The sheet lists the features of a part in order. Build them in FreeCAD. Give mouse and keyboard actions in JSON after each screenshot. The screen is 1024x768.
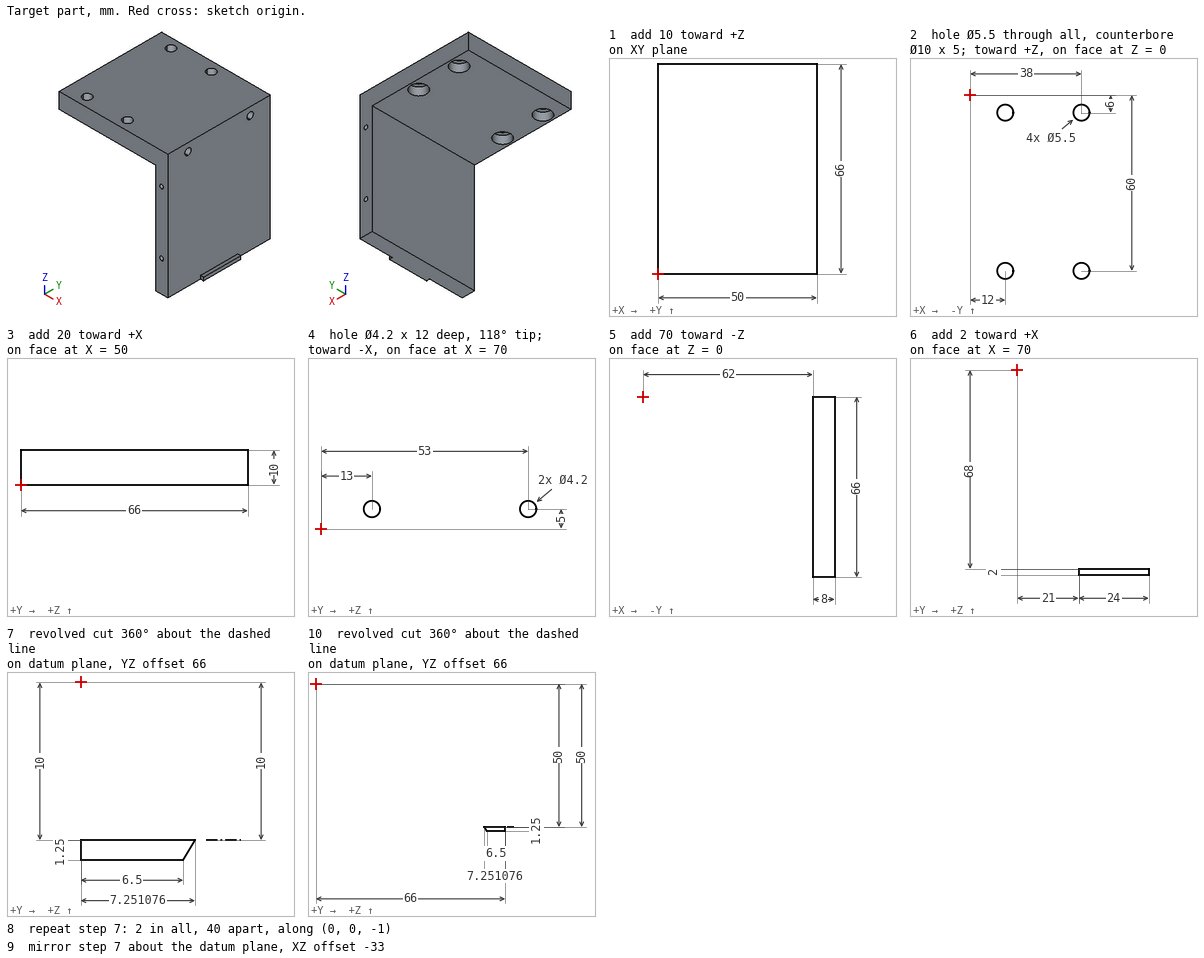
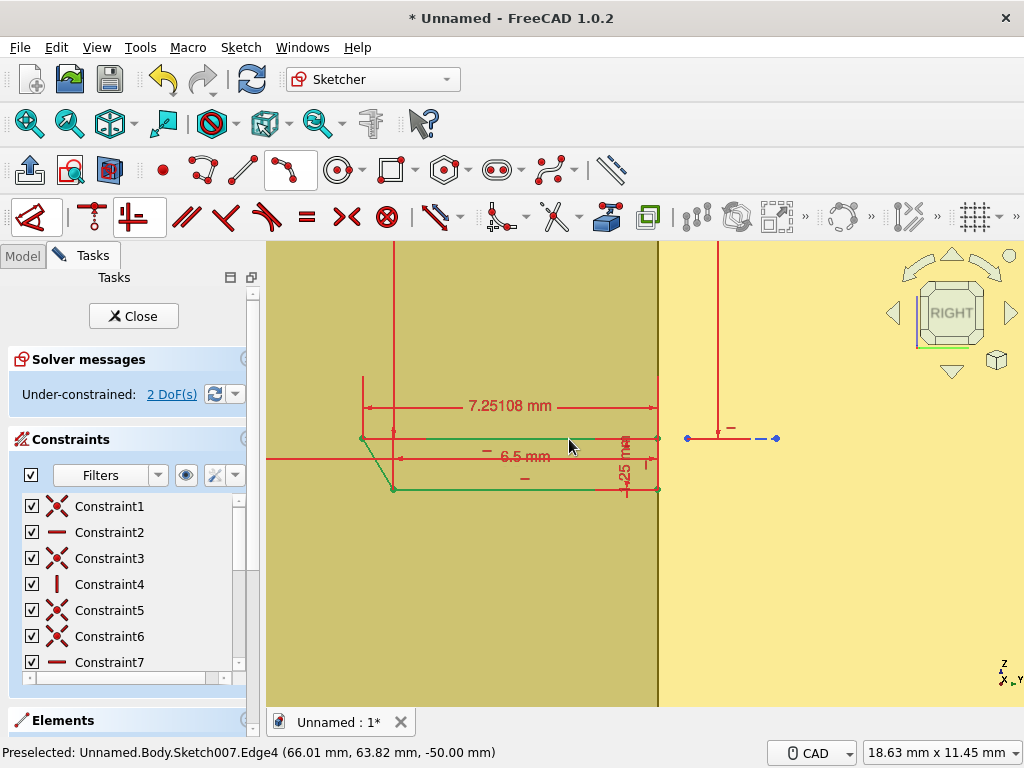
{"action": "left_click", "coordinate": [134, 316]}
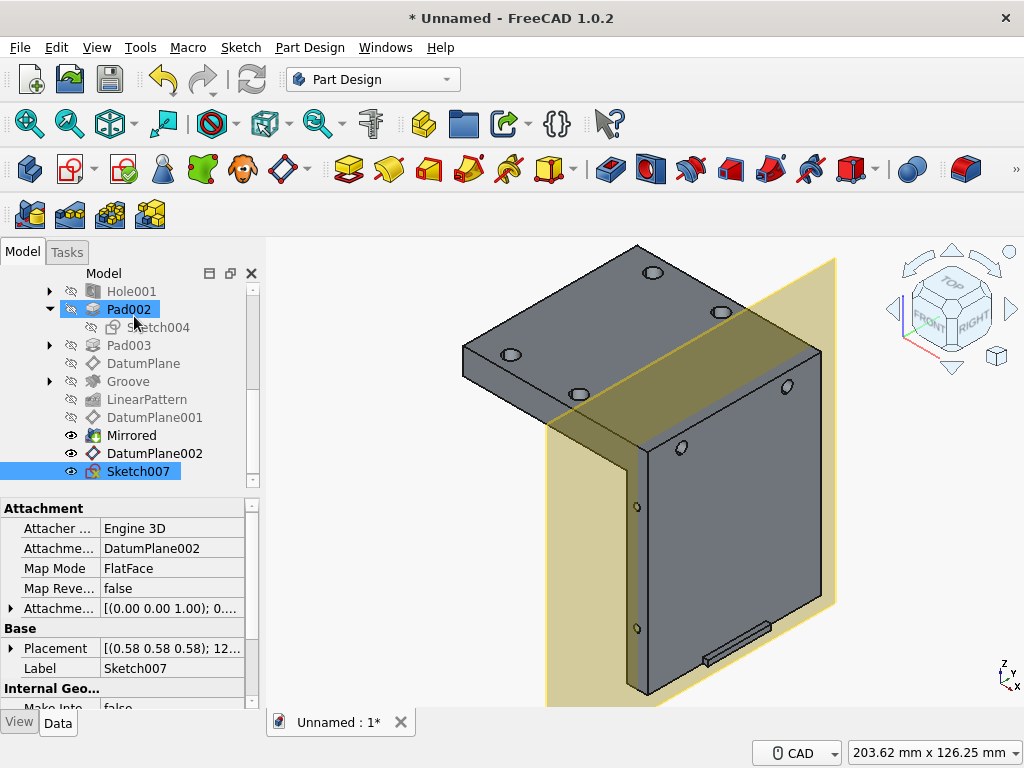
{"action": "left_click", "coordinate": [692, 170]}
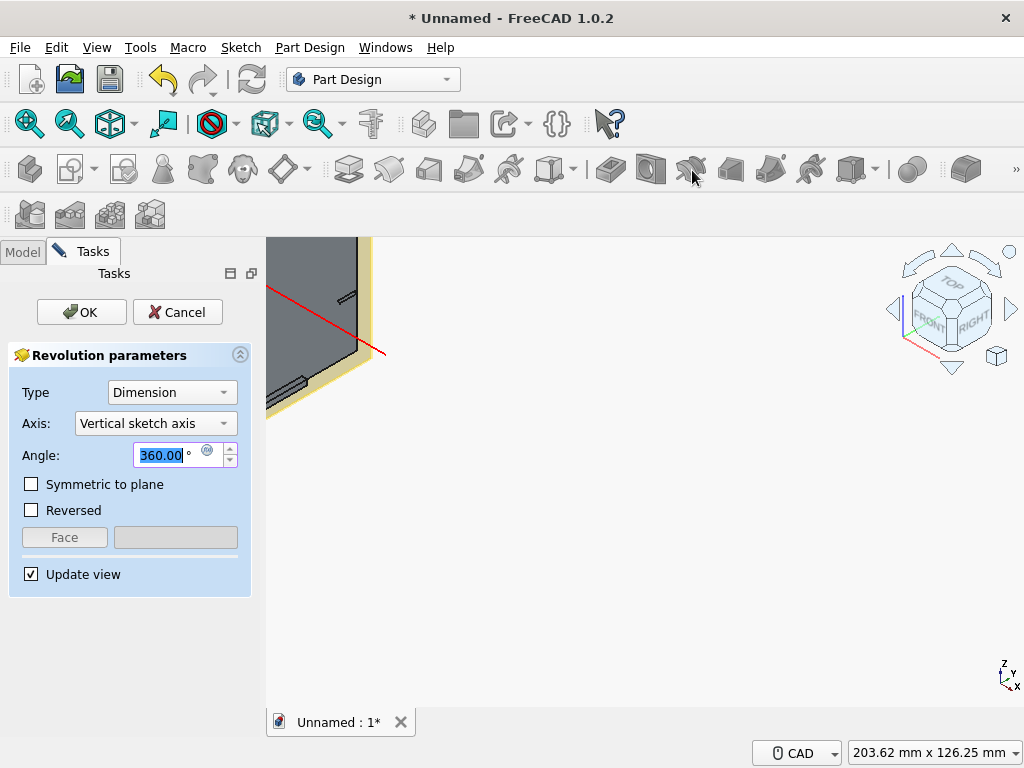
{"action": "left_click", "coordinate": [156, 424]}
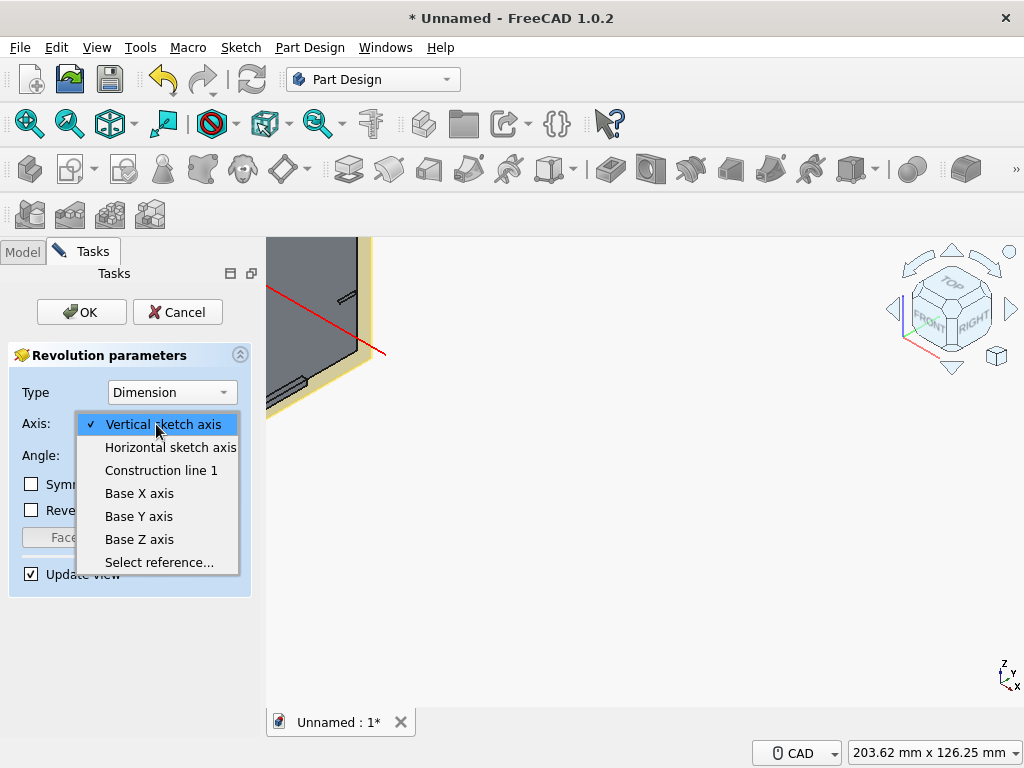
{"action": "left_click", "coordinate": [156, 470]}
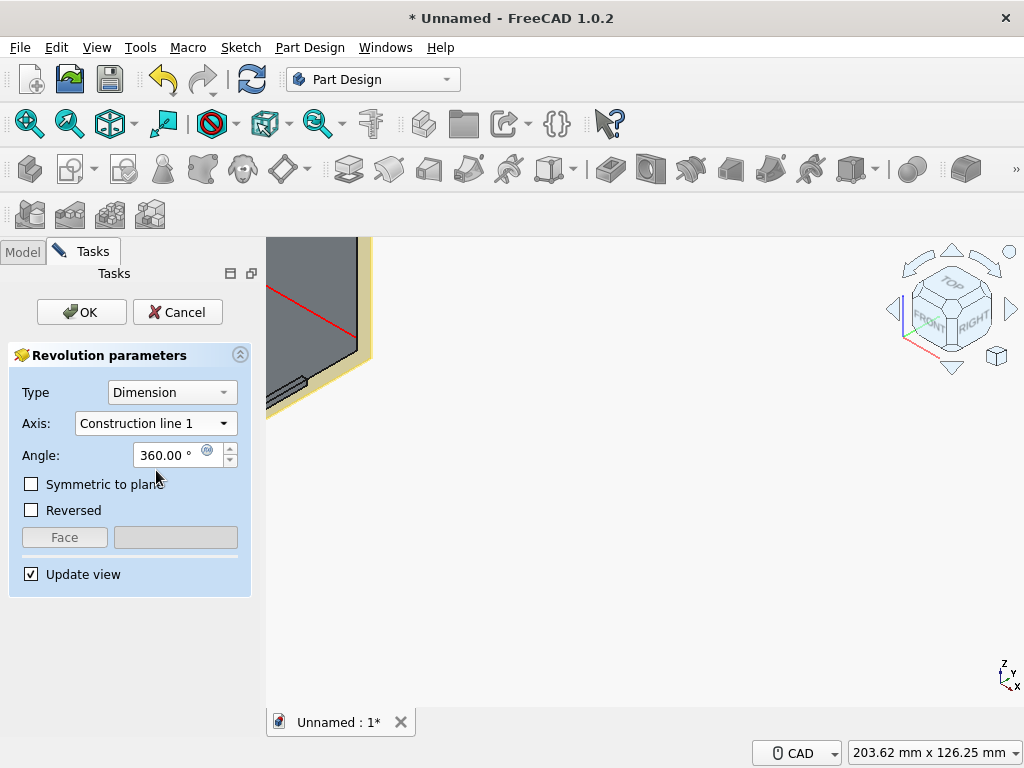
{"action": "left_click", "coordinate": [82, 312]}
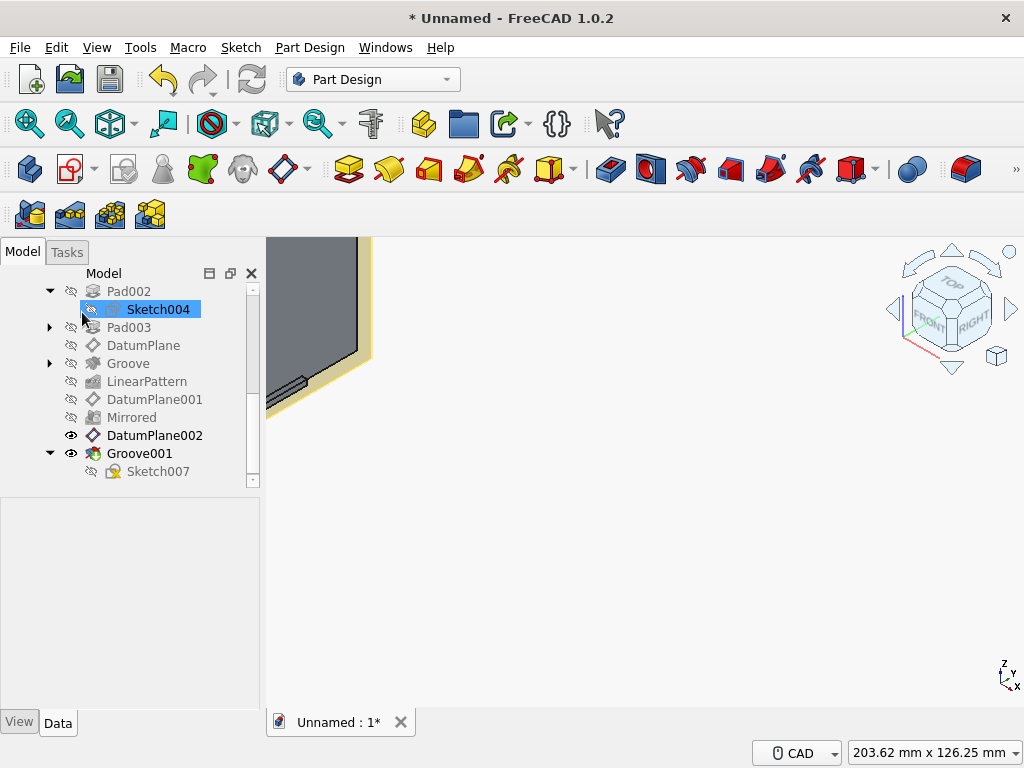
{"action": "left_click", "coordinate": [116, 435]}
{"action": "key", "text": "space"}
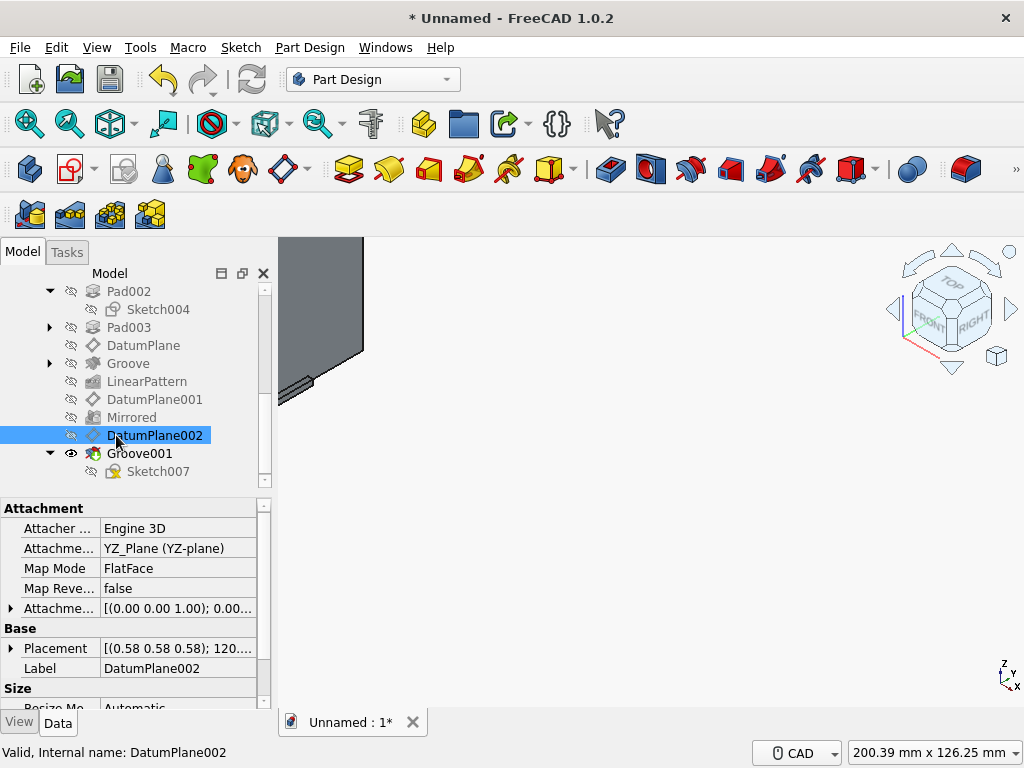
{"action": "key", "text": "v f"}